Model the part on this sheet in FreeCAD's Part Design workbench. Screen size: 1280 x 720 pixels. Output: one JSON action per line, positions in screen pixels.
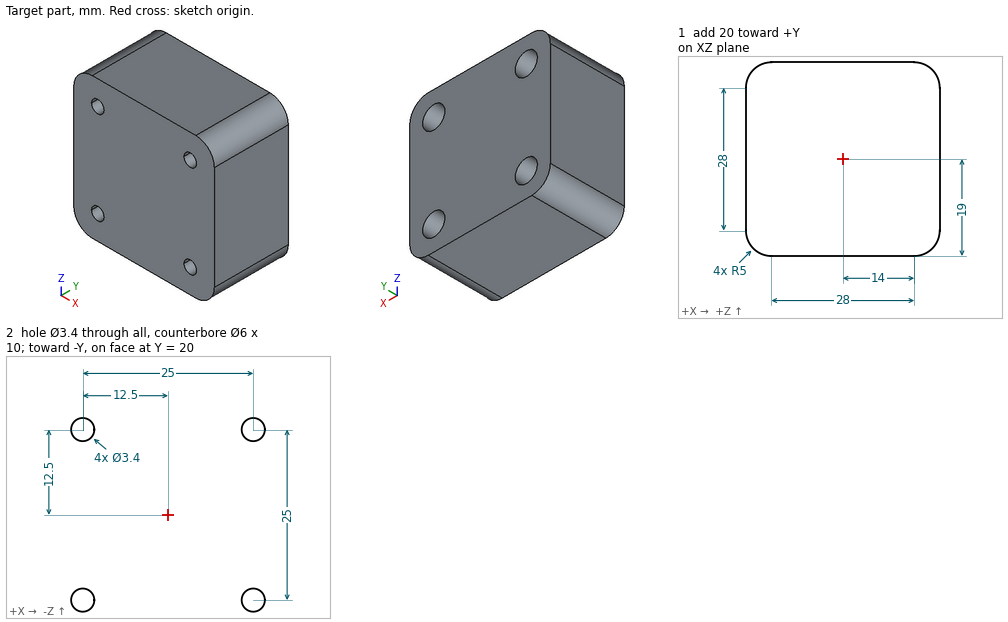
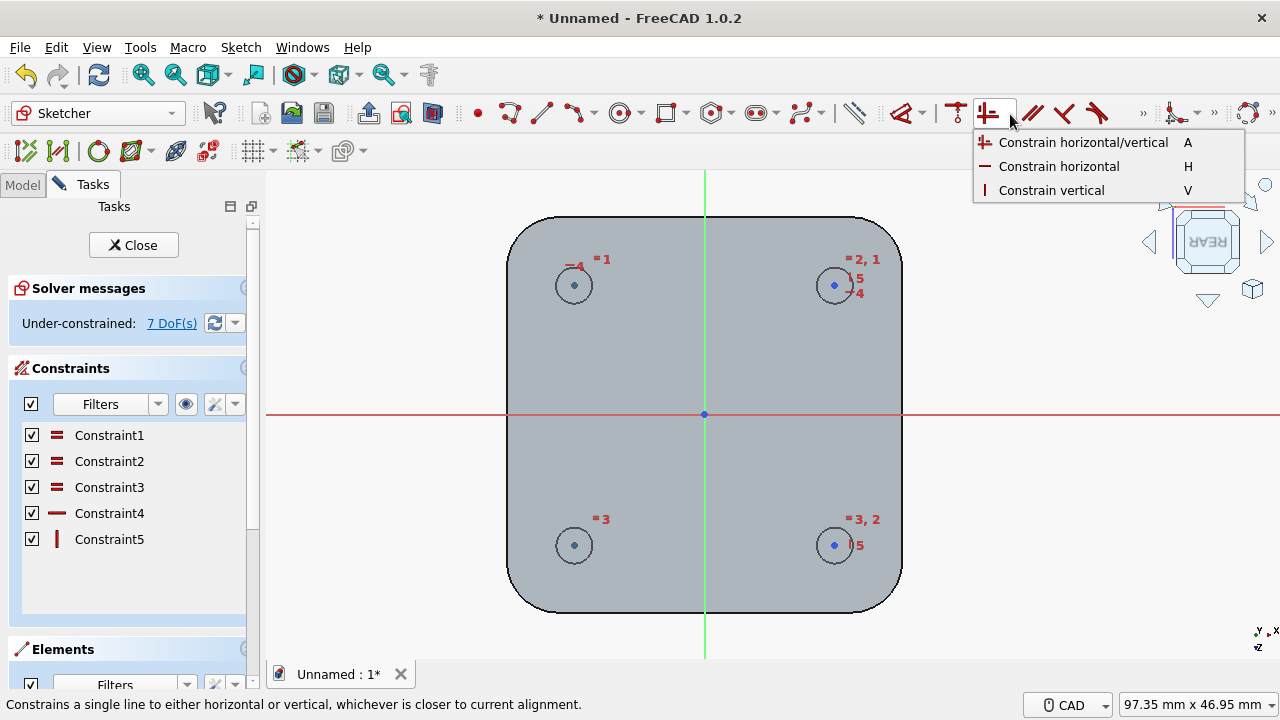
{"action": "left_click", "coordinate": [1109, 190]}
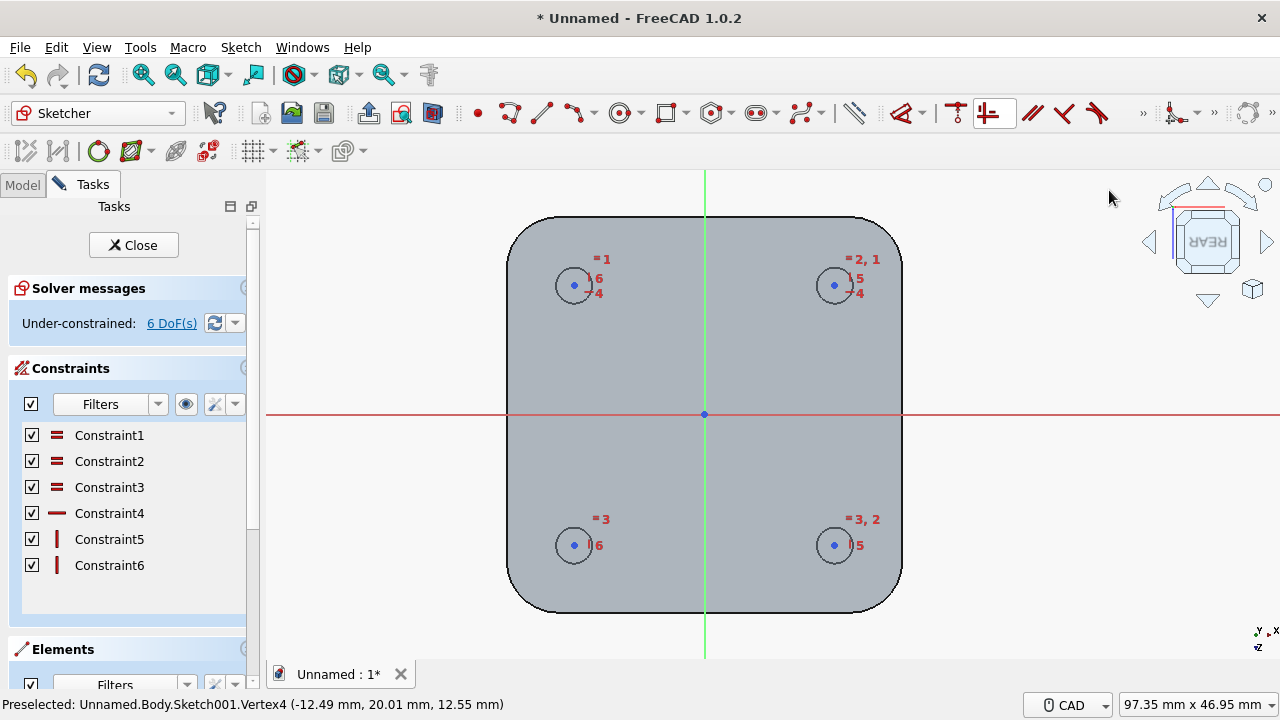
{"action": "left_click", "coordinate": [835, 546]}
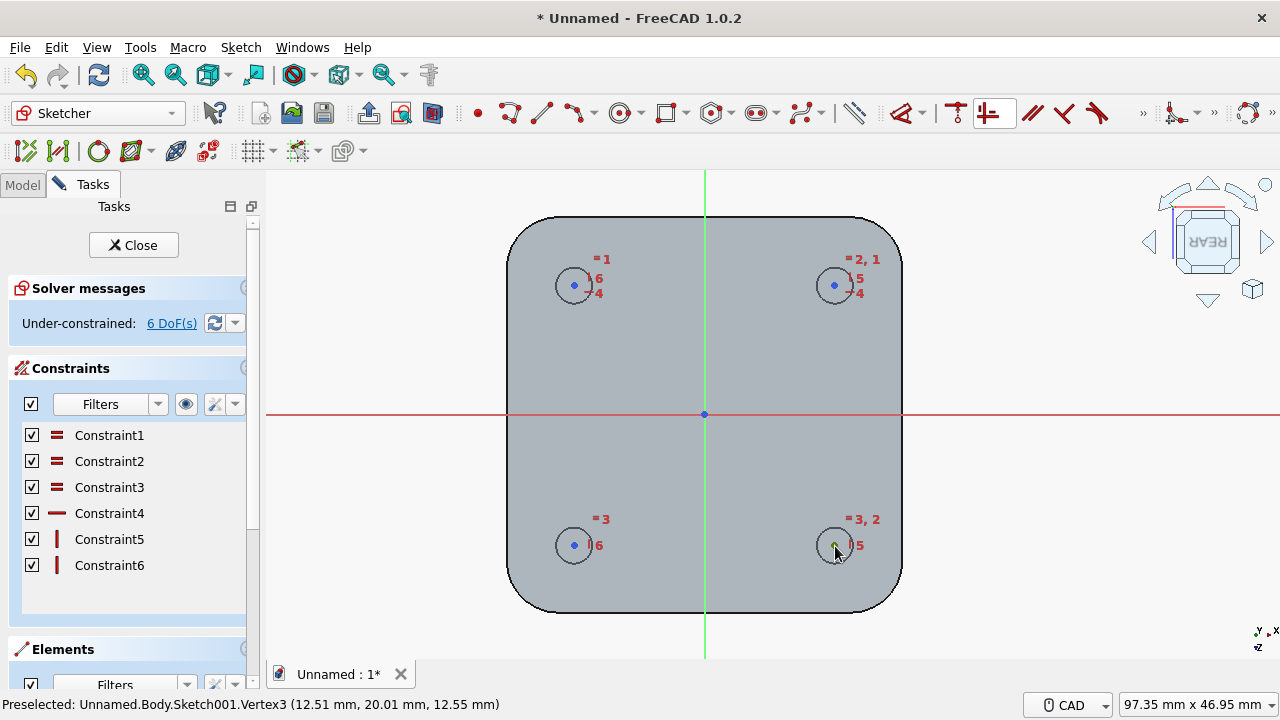
{"action": "left_click", "coordinate": [574, 546]}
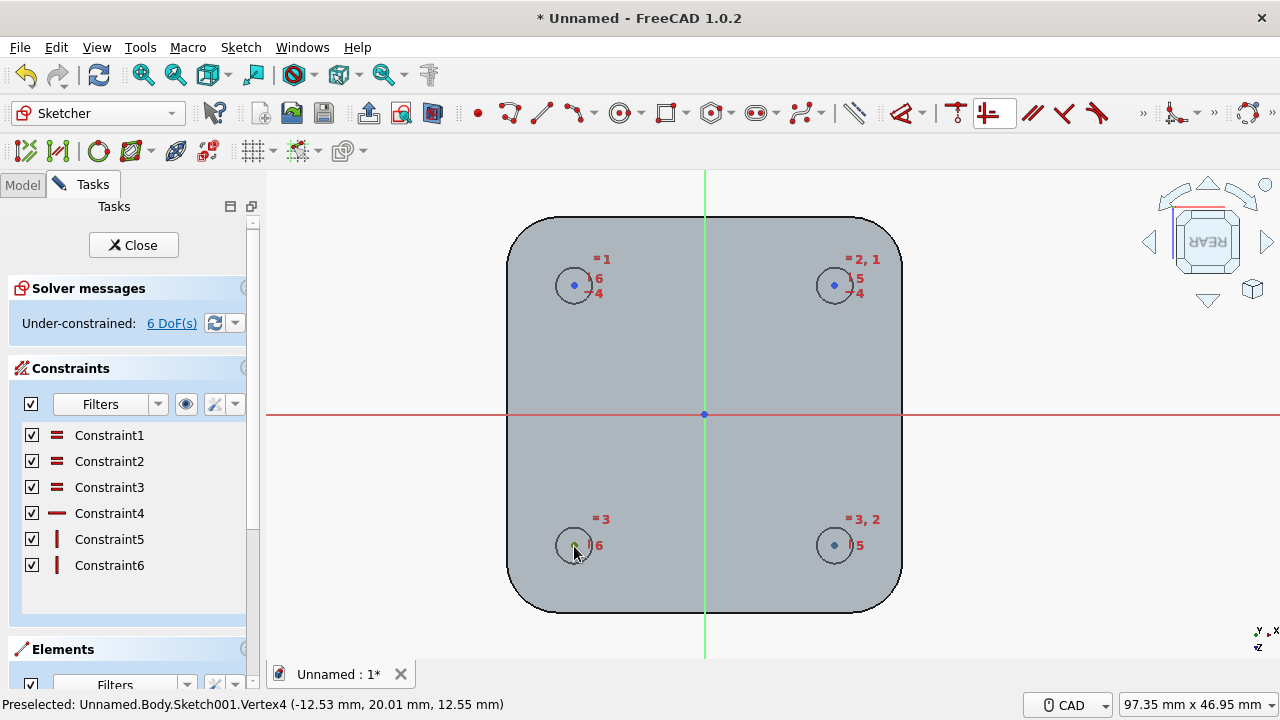
{"action": "left_click", "coordinate": [1010, 114]}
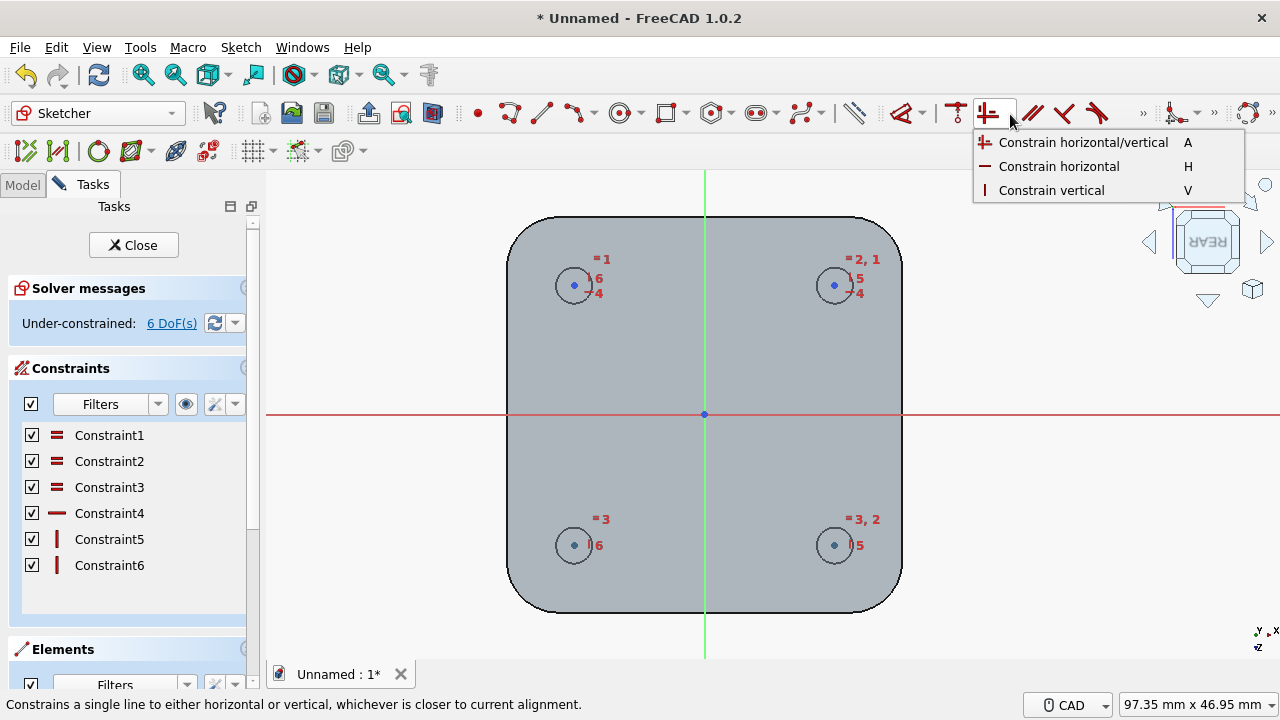
{"action": "left_click", "coordinate": [1109, 166]}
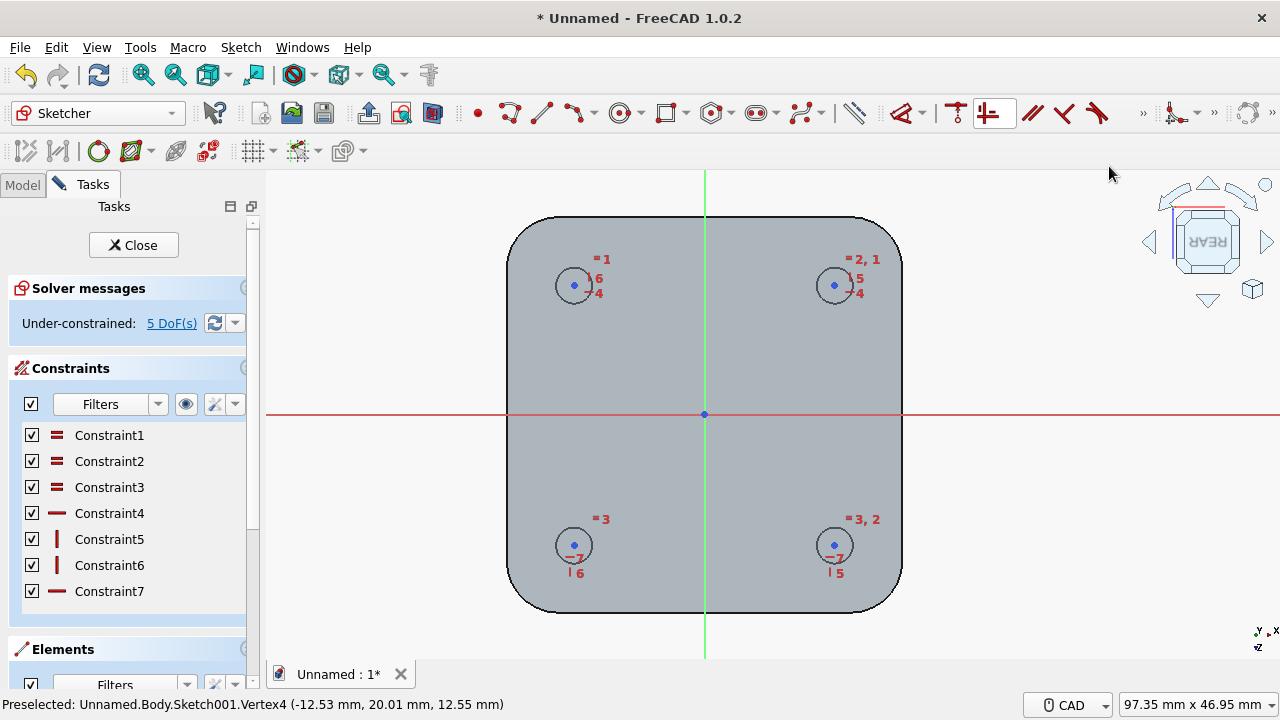
{"action": "left_click", "coordinate": [902, 114]}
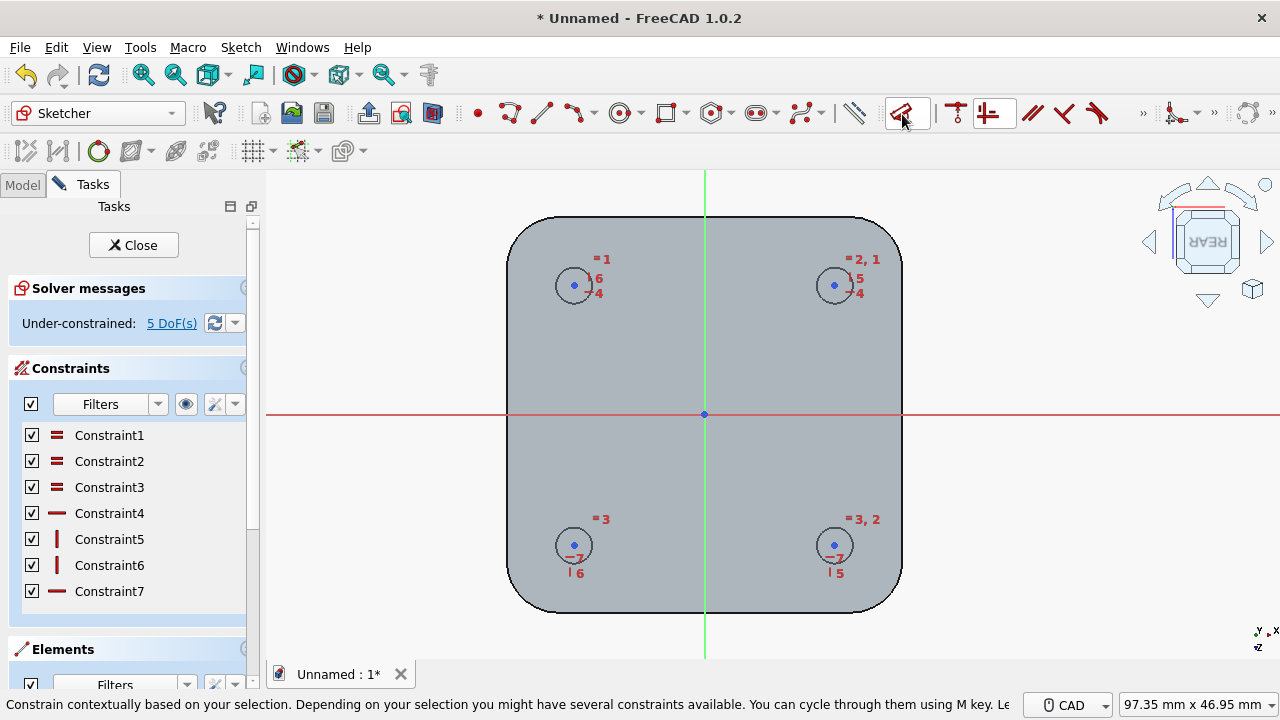
{"action": "left_click", "coordinate": [587, 273]}
{"action": "left_click", "coordinate": [610, 251]}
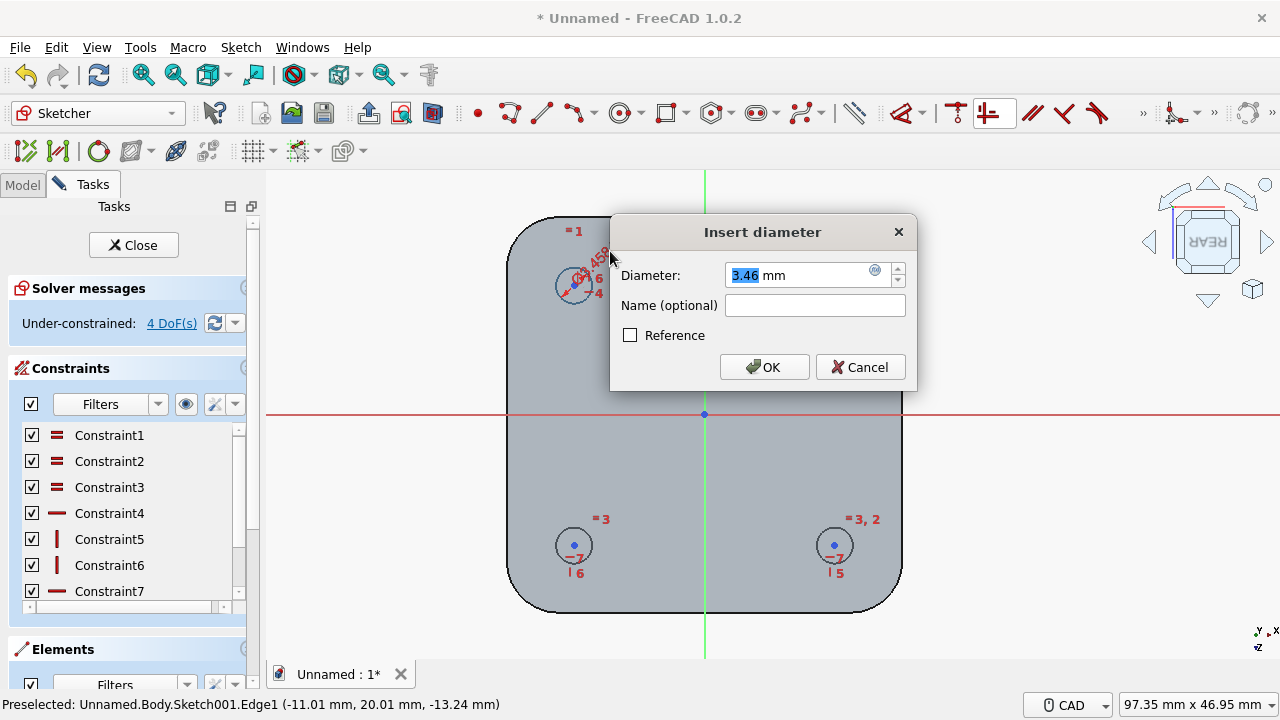
{"action": "type", "text": "3.4"}
{"action": "key", "text": "Return"}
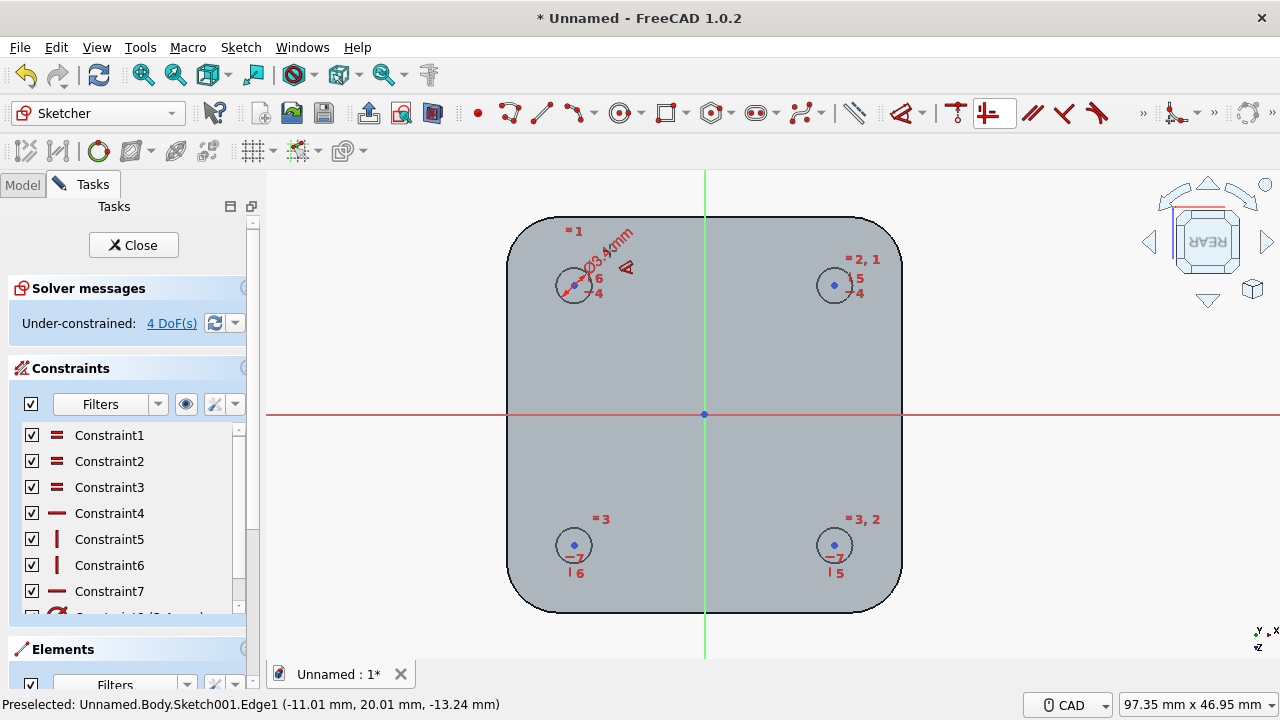
{"action": "left_click", "coordinate": [574, 286]}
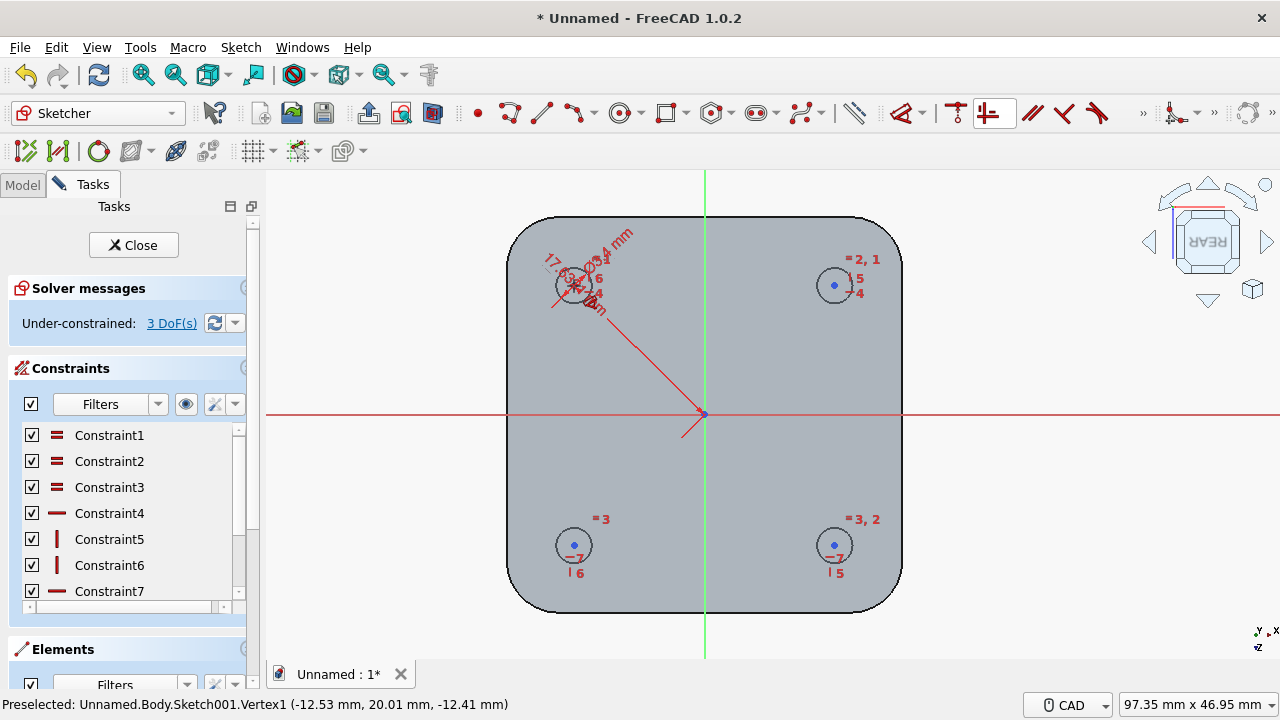
{"action": "left_click", "coordinate": [835, 286]}
{"action": "left_click", "coordinate": [764, 252]}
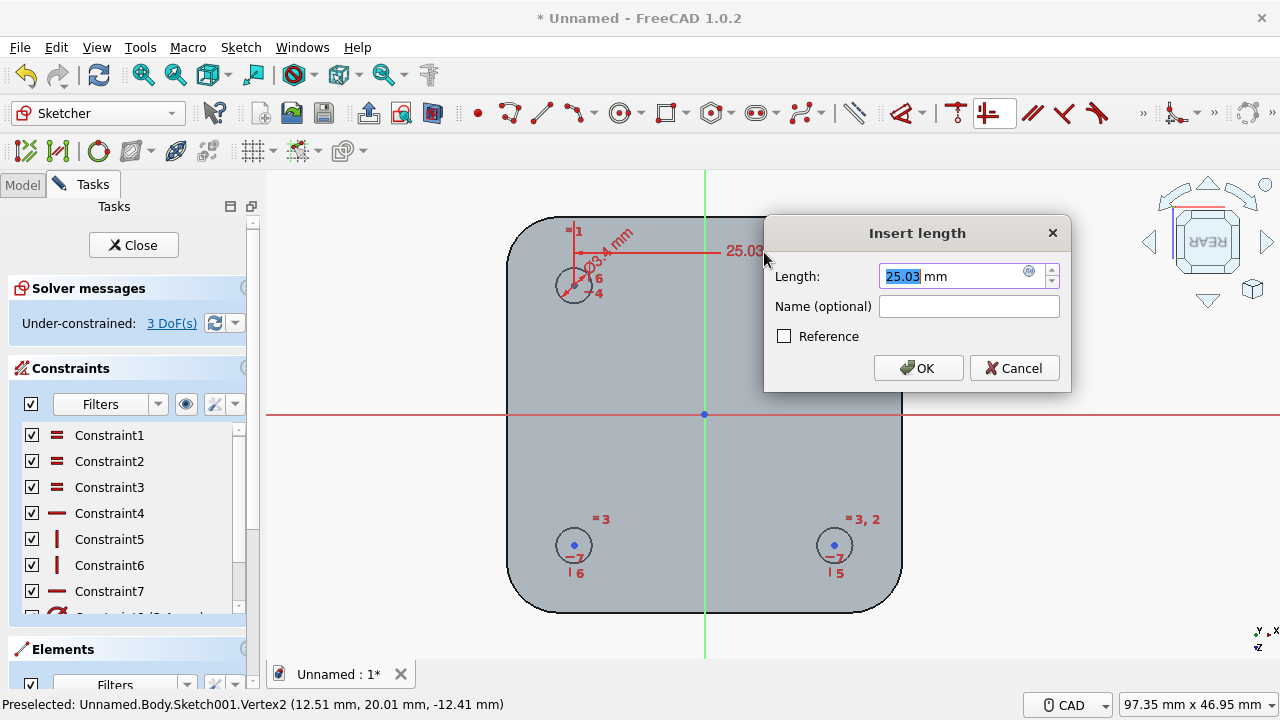
{"action": "type", "text": "25"}
{"action": "key", "text": "Return"}